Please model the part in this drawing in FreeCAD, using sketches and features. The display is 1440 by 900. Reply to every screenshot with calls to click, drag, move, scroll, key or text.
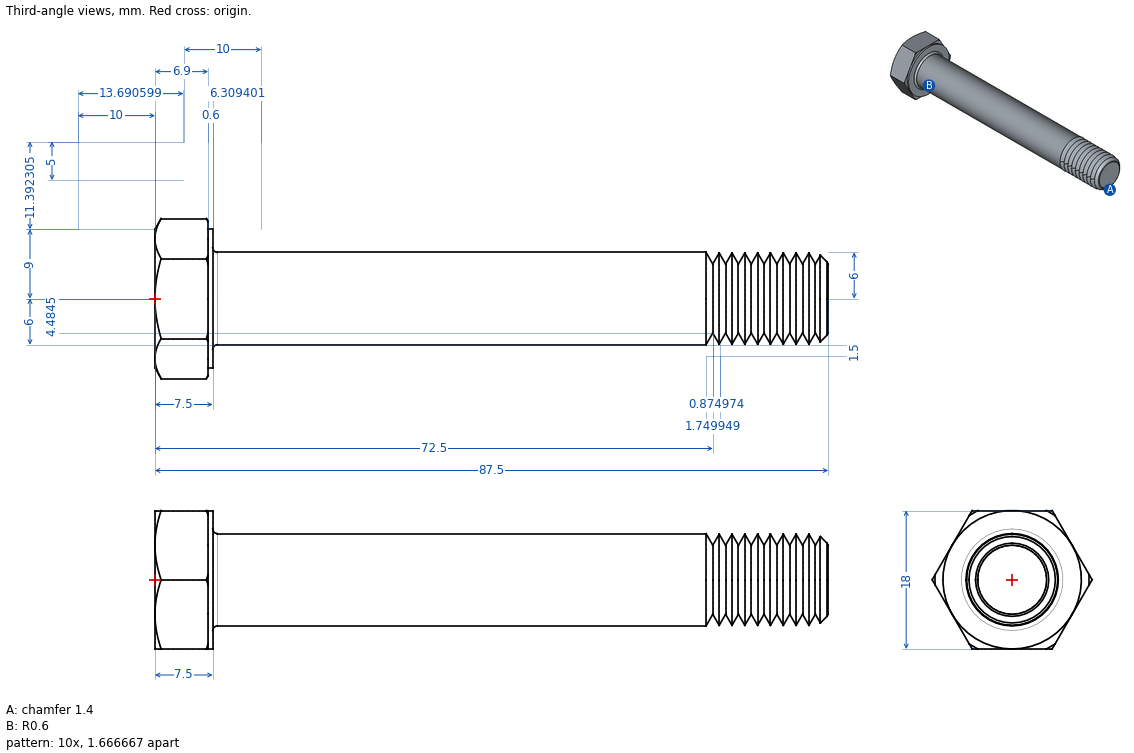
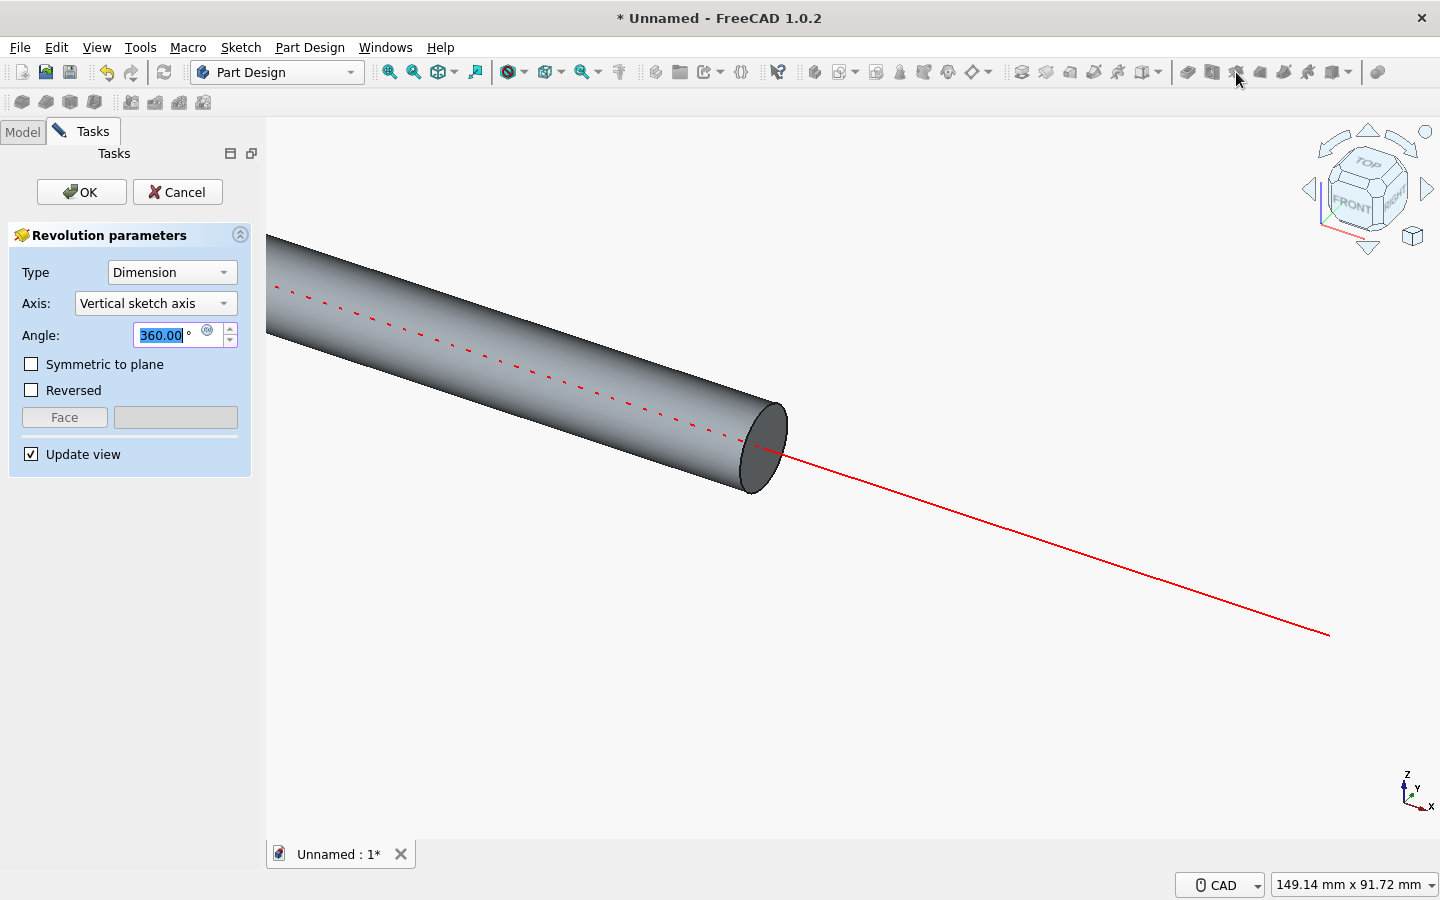
click(156, 304)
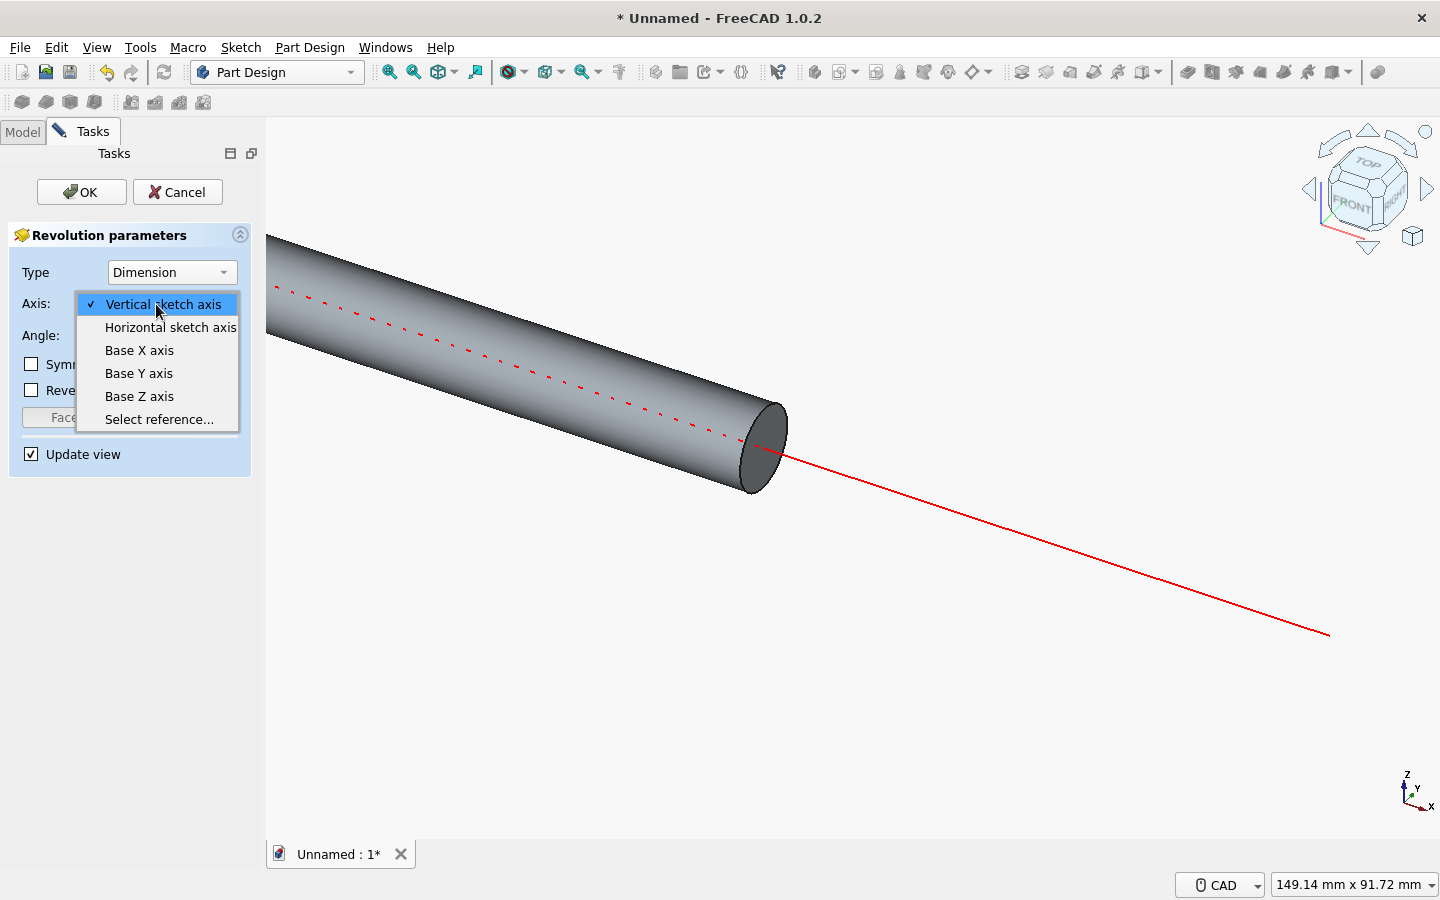
click(156, 328)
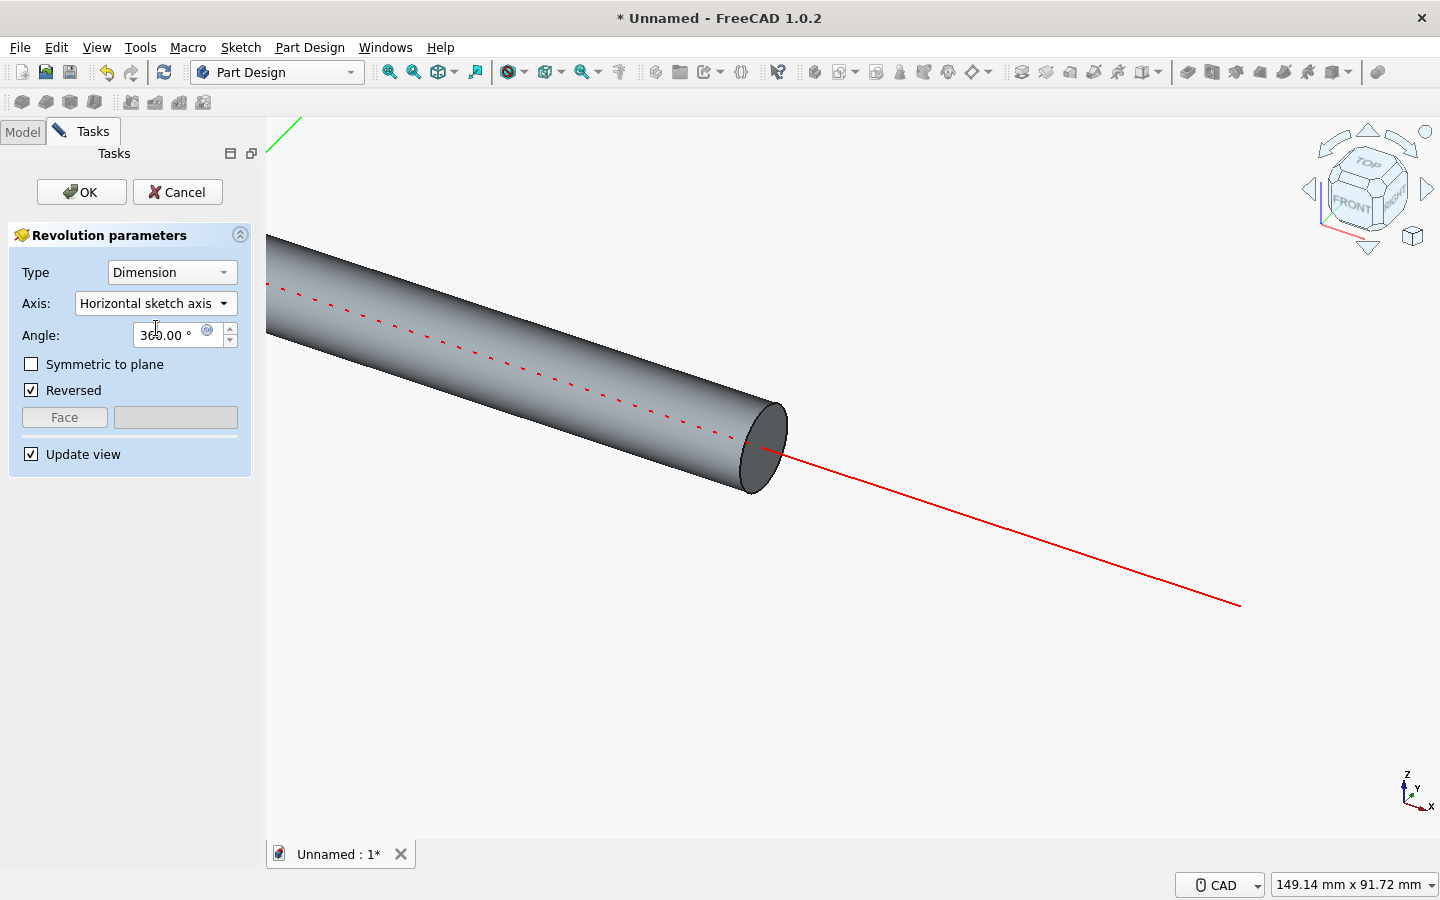
click(82, 192)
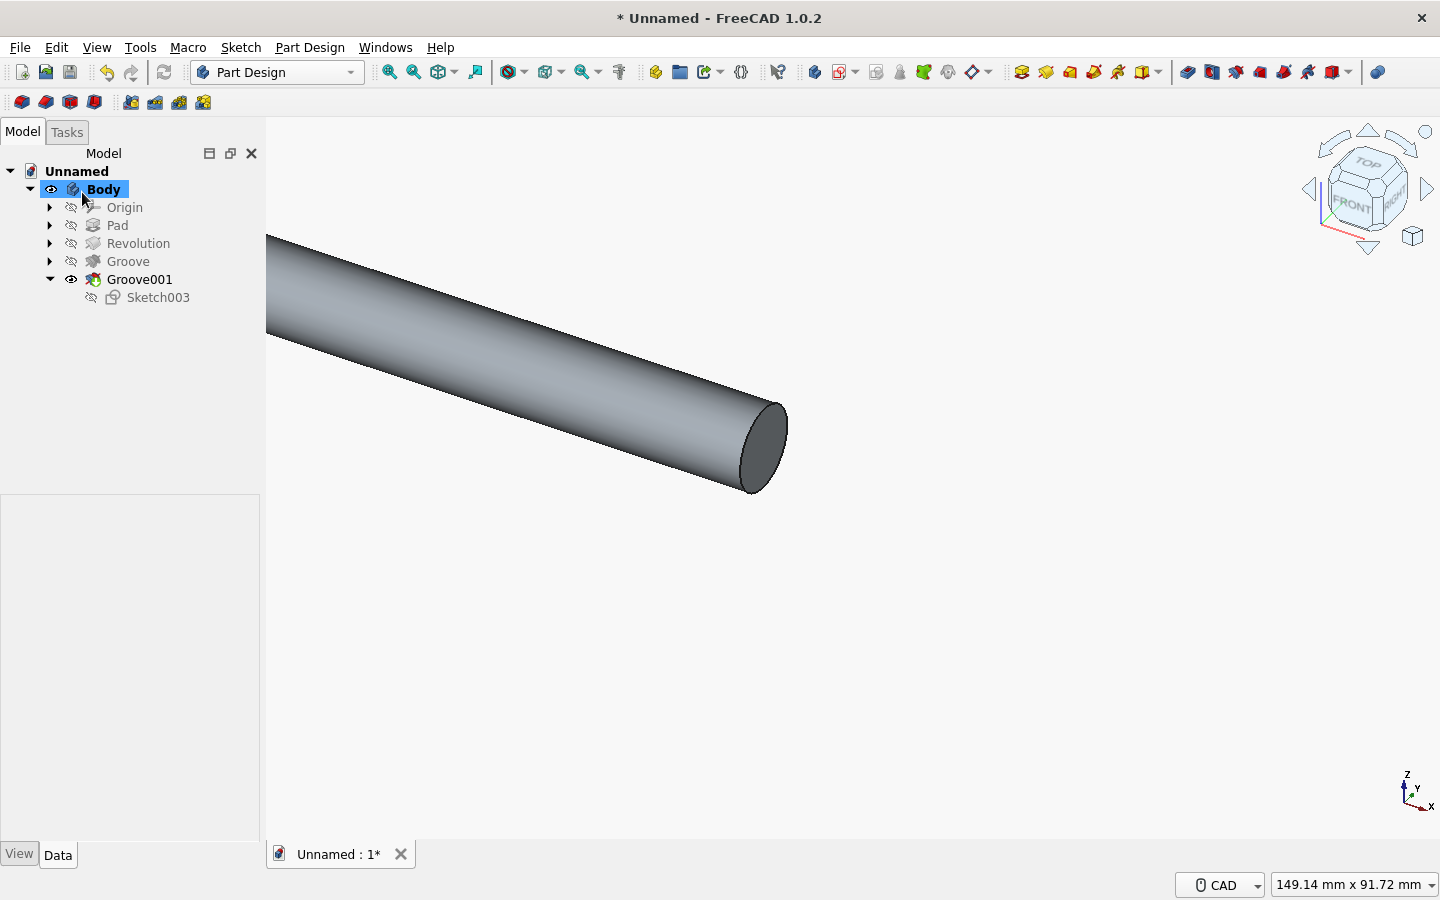
click(390, 72)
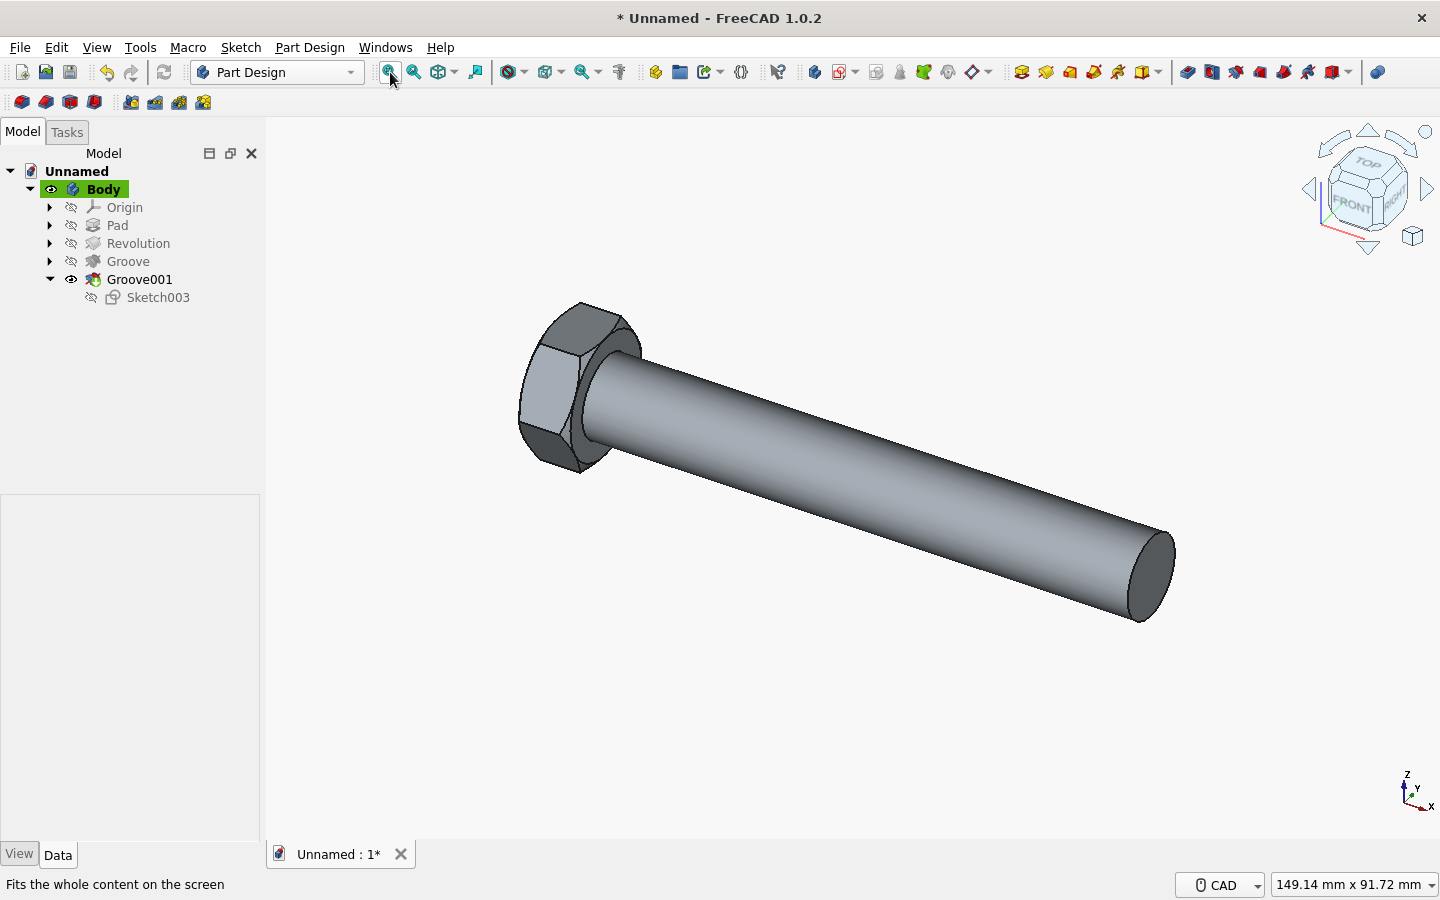
click(840, 72)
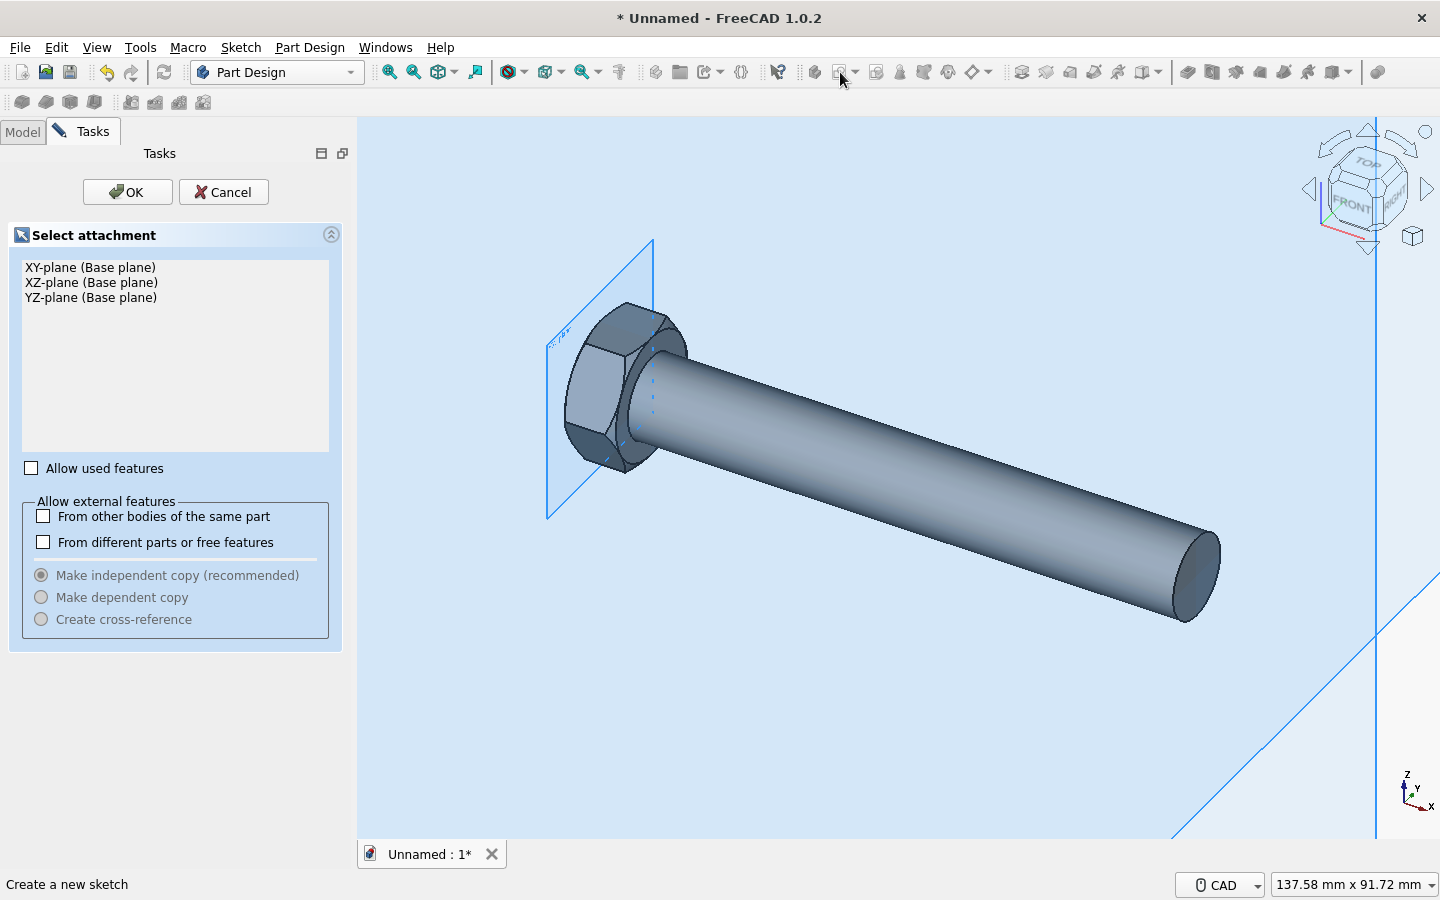
click(82, 268)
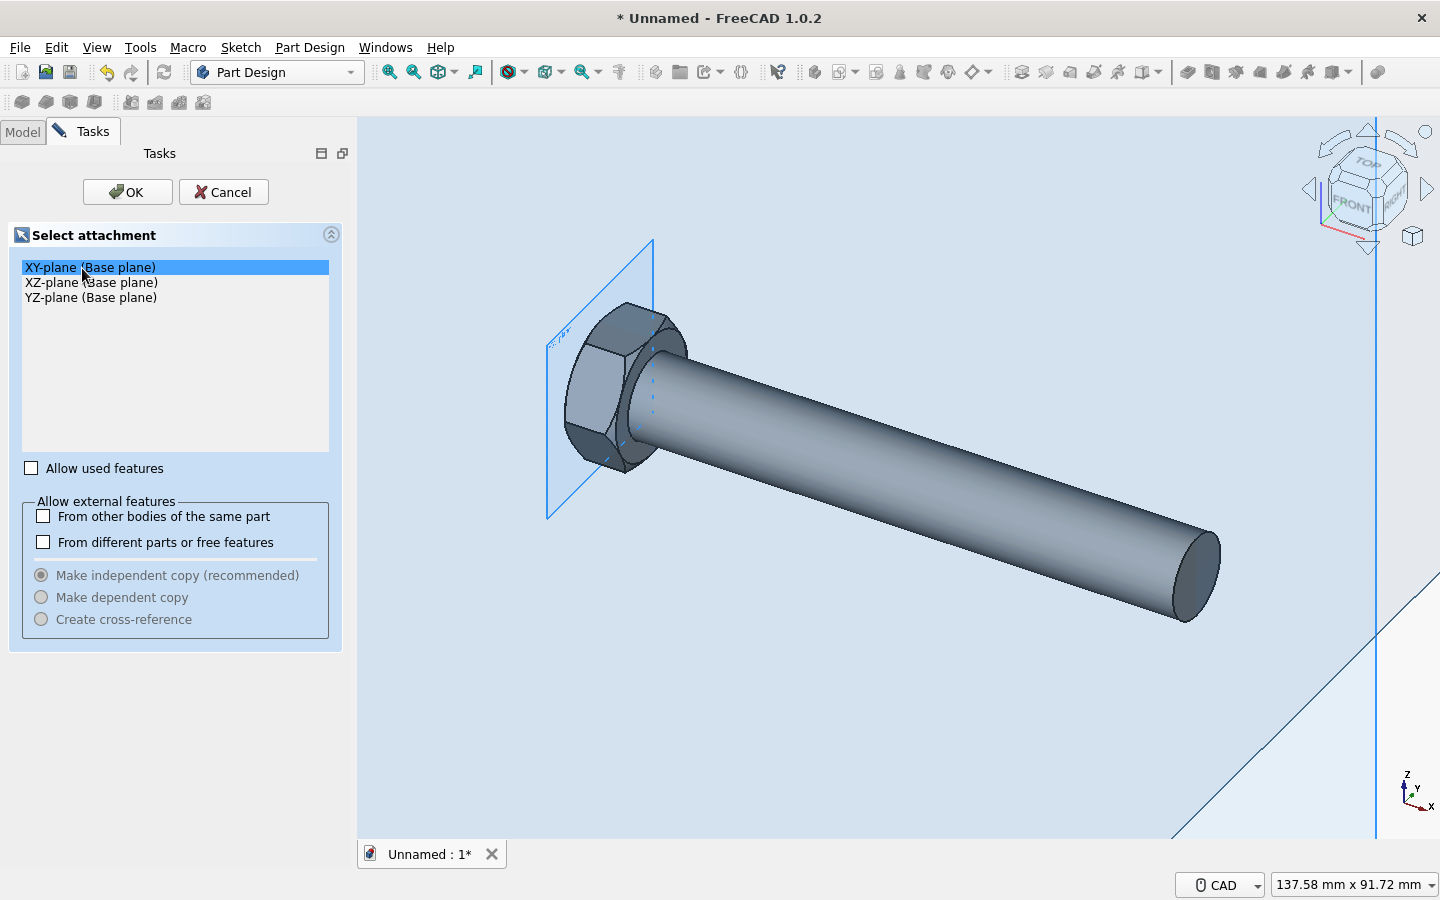
click(128, 192)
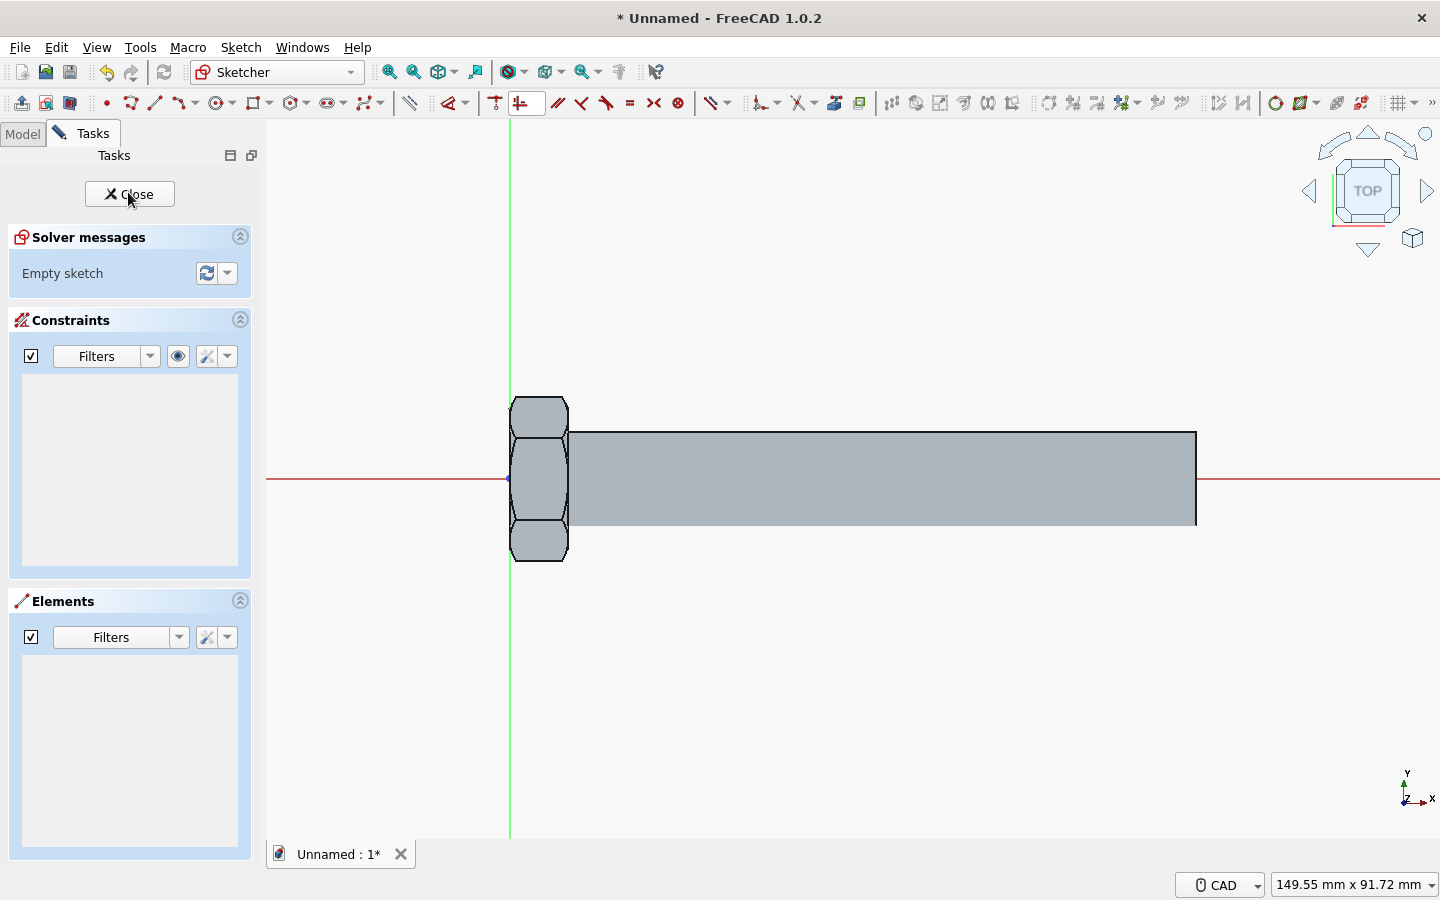
click(70, 104)